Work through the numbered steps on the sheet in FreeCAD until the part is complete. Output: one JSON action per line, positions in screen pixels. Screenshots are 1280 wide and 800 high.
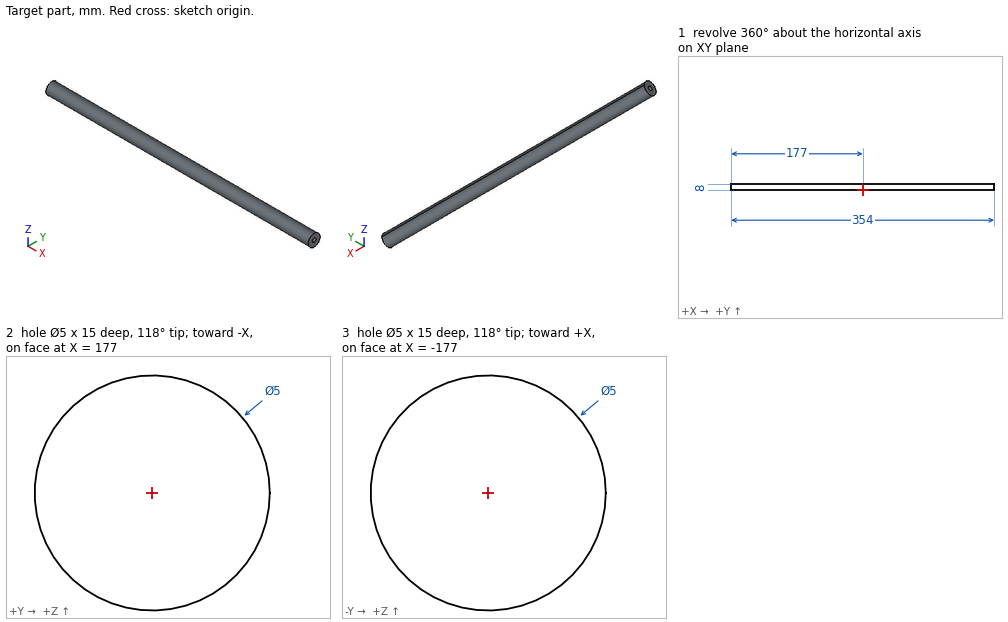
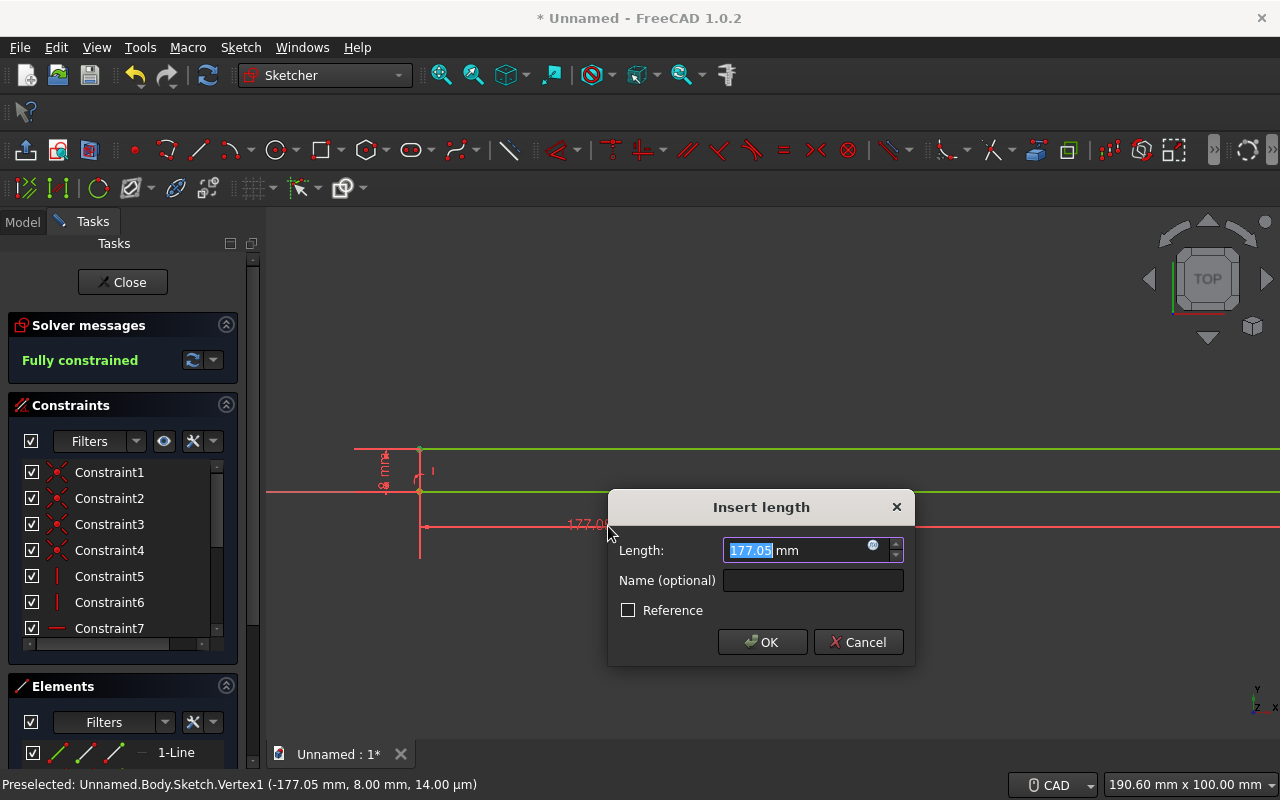
{"action": "type", "text": "177"}
{"action": "key", "text": "Return"}
{"action": "key", "text": "Escape"}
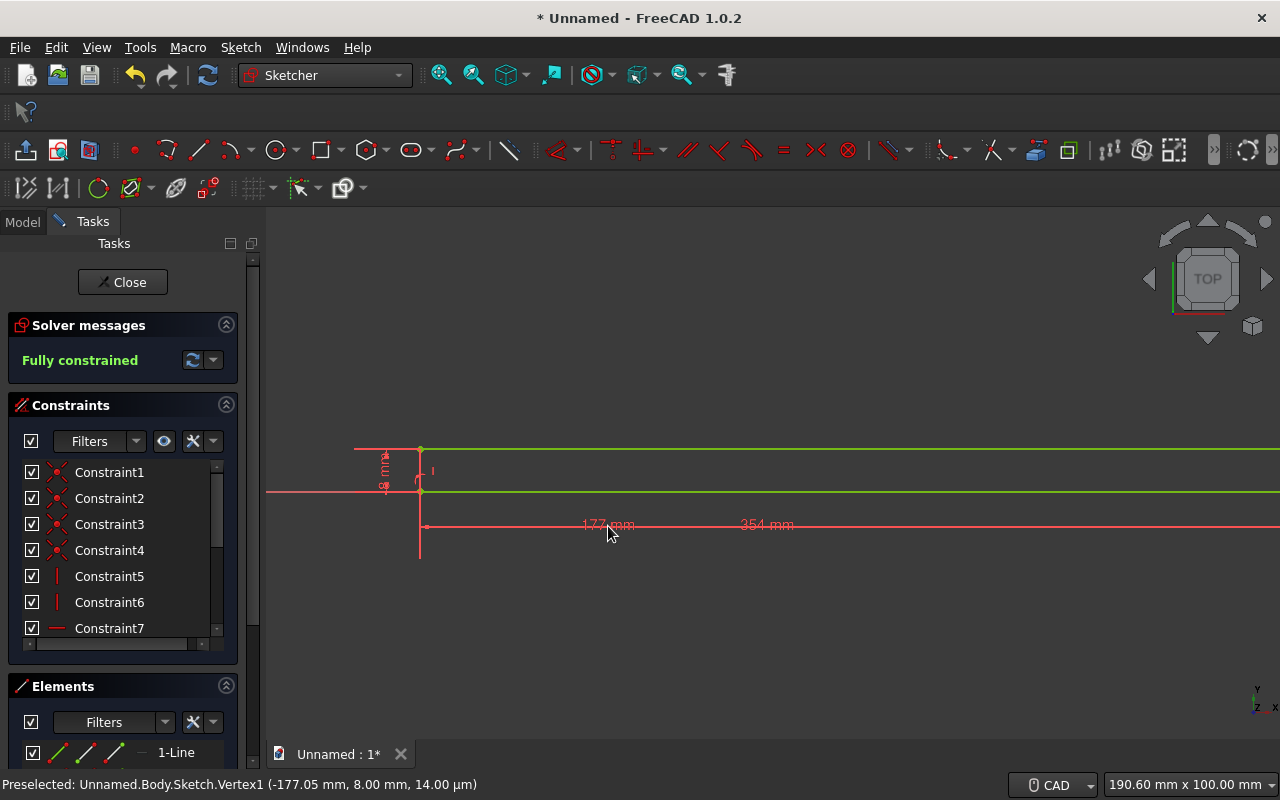
{"action": "left_click", "coordinate": [123, 282]}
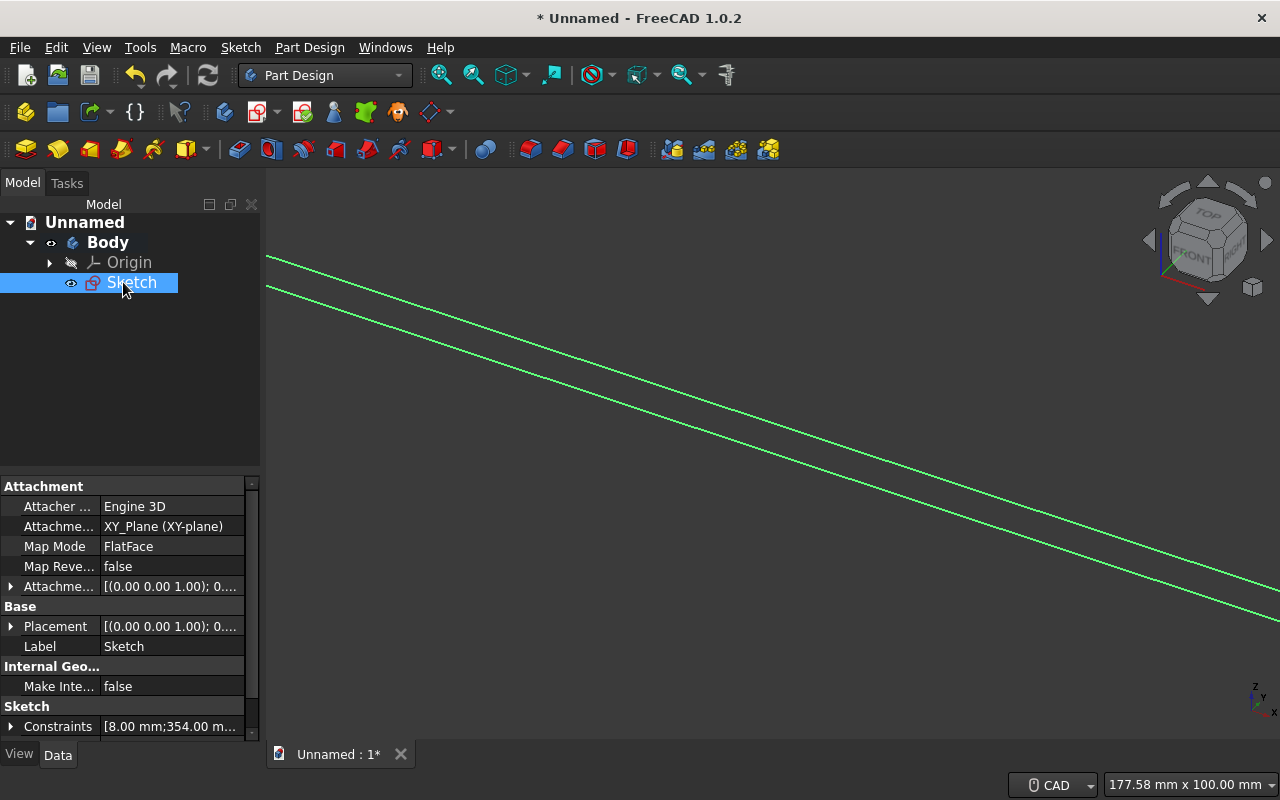
{"action": "left_click", "coordinate": [58, 150]}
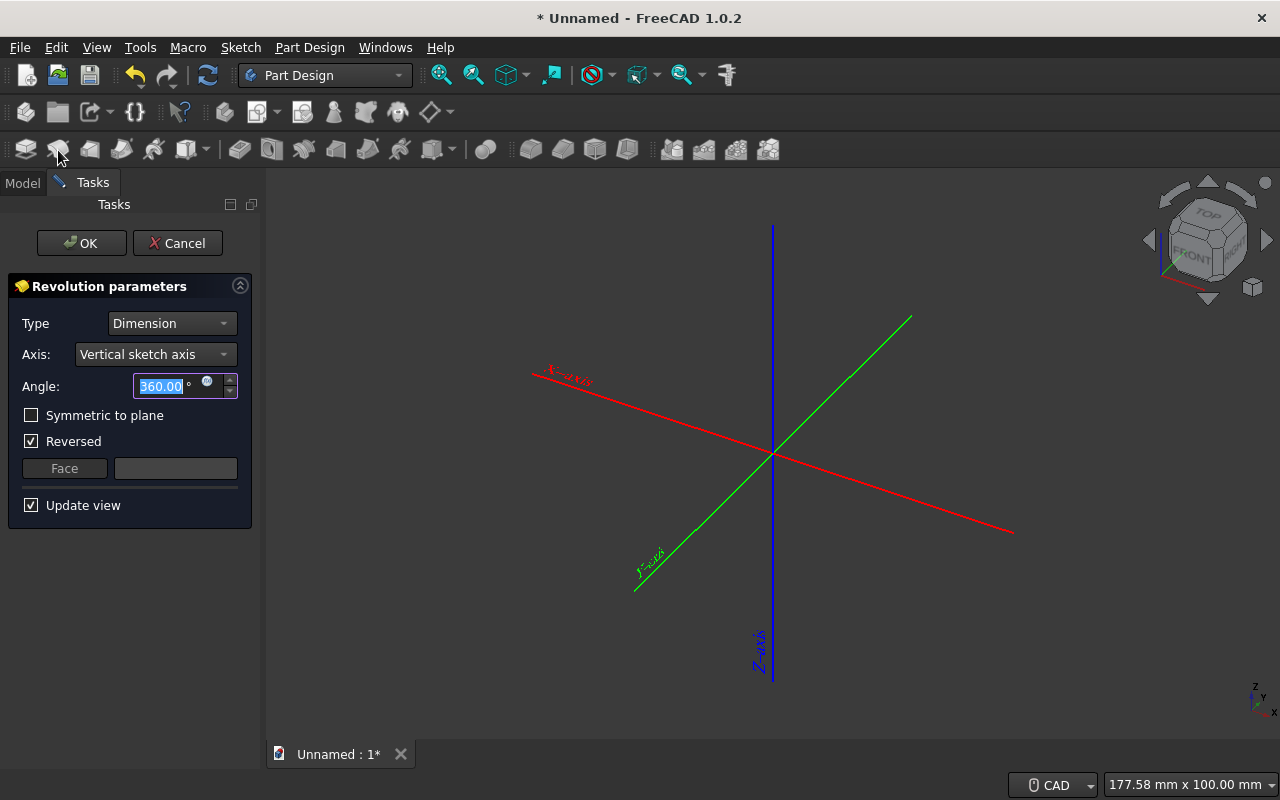
{"action": "left_click", "coordinate": [156, 354]}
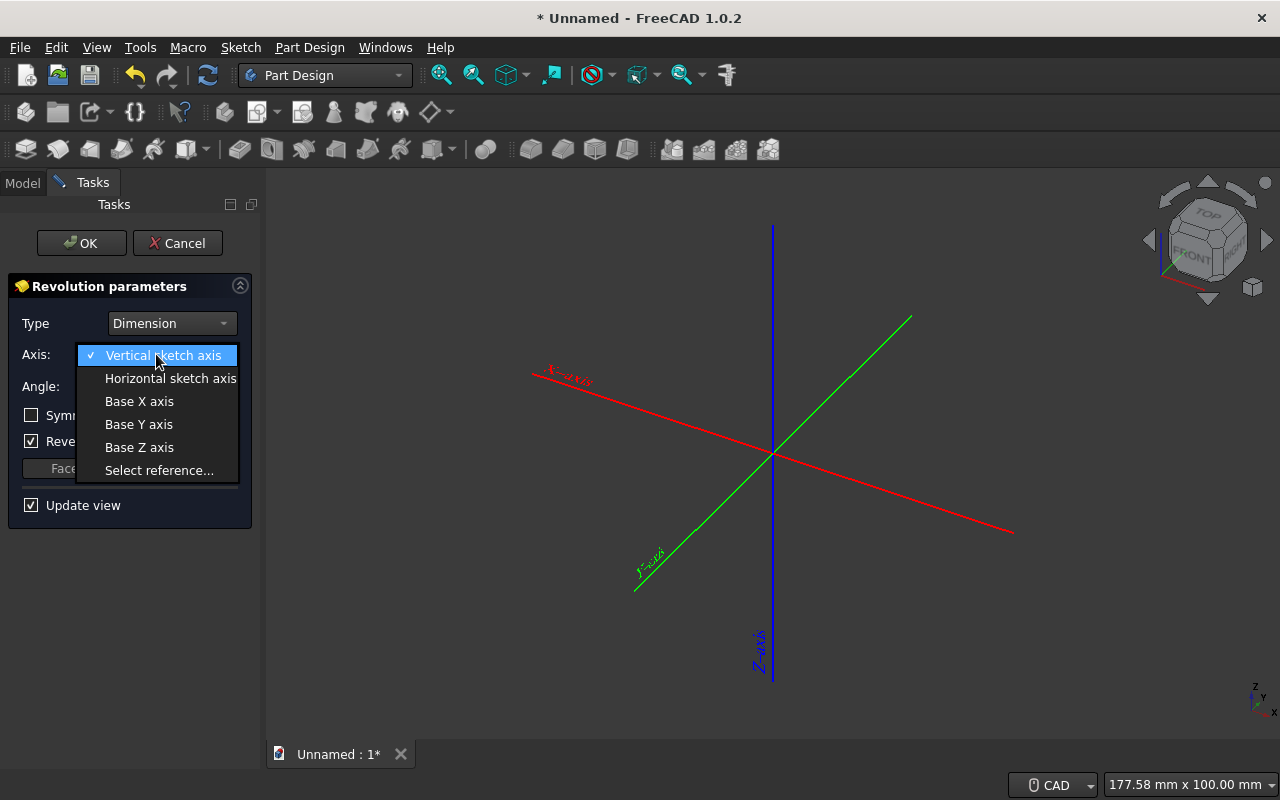
{"action": "left_click", "coordinate": [156, 378]}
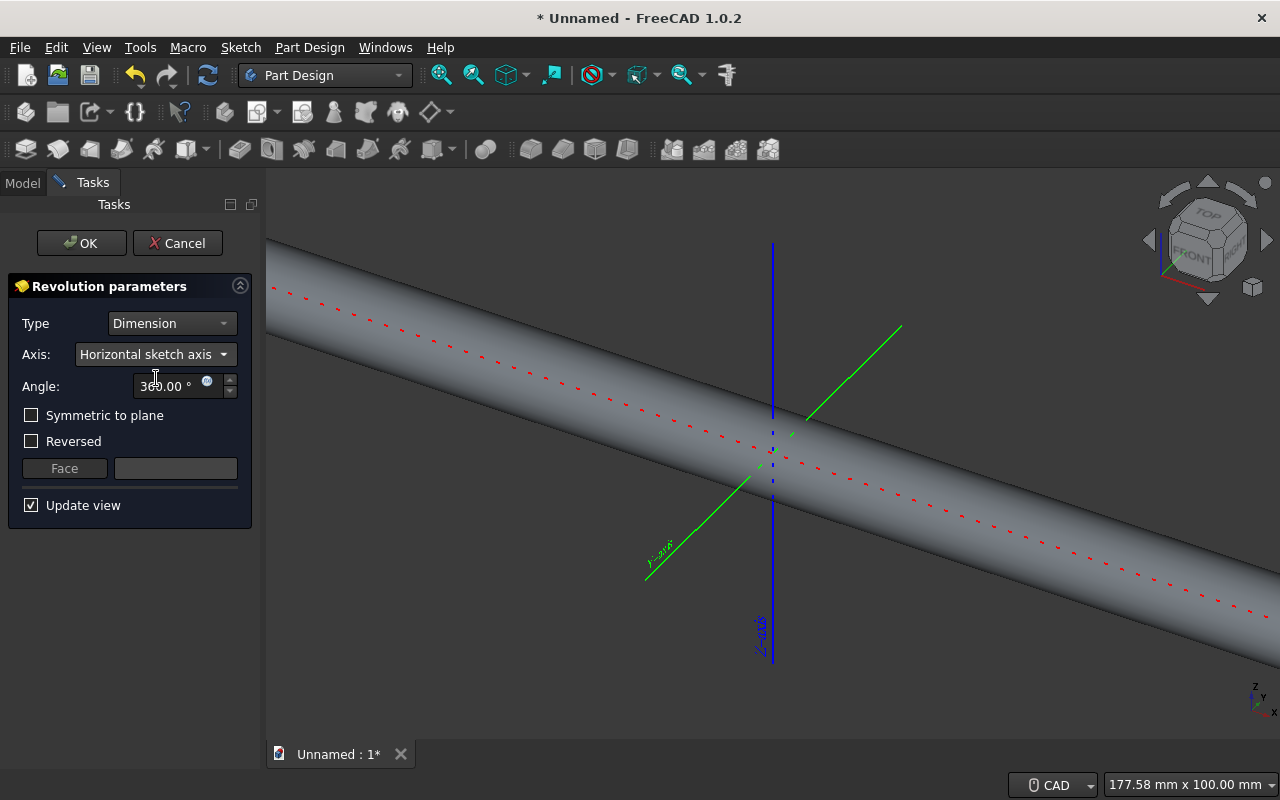
{"action": "left_click", "coordinate": [82, 243]}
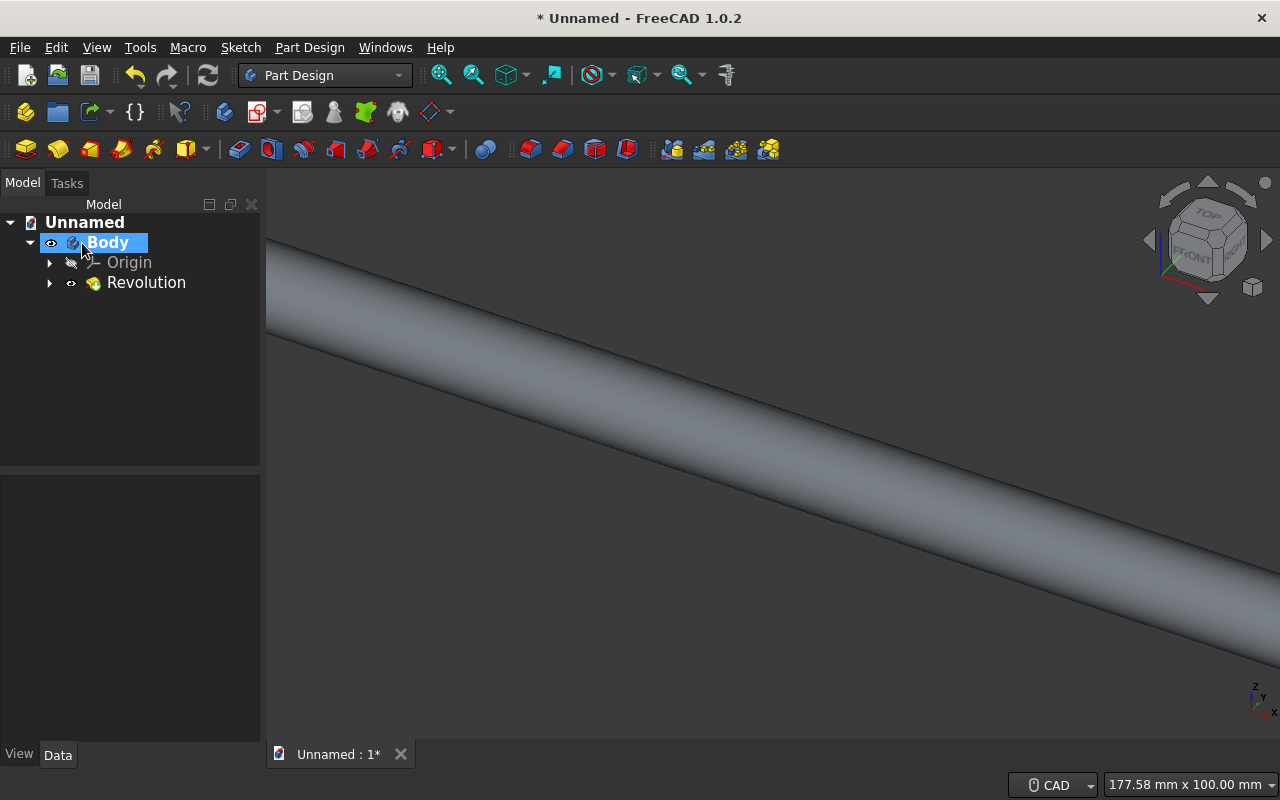
{"action": "left_click", "coordinate": [442, 76]}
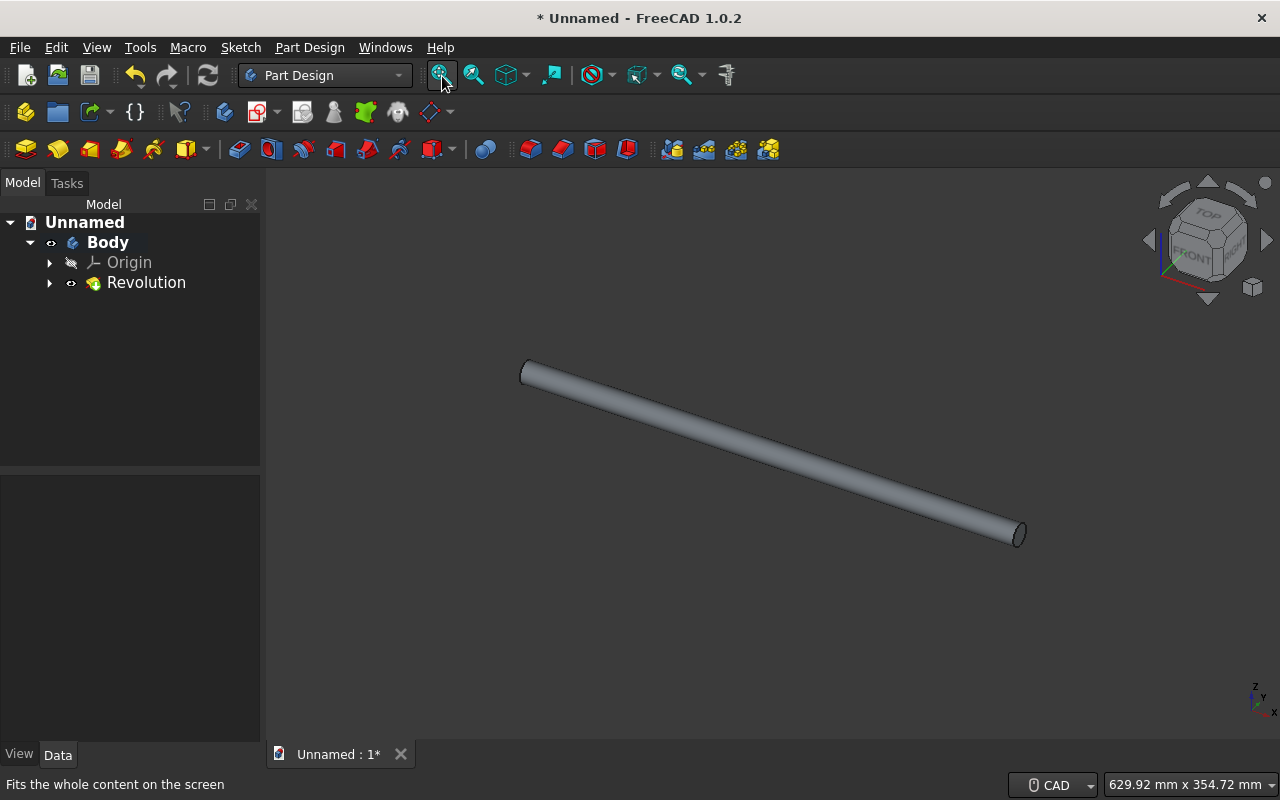
{"action": "key", "text": "0"}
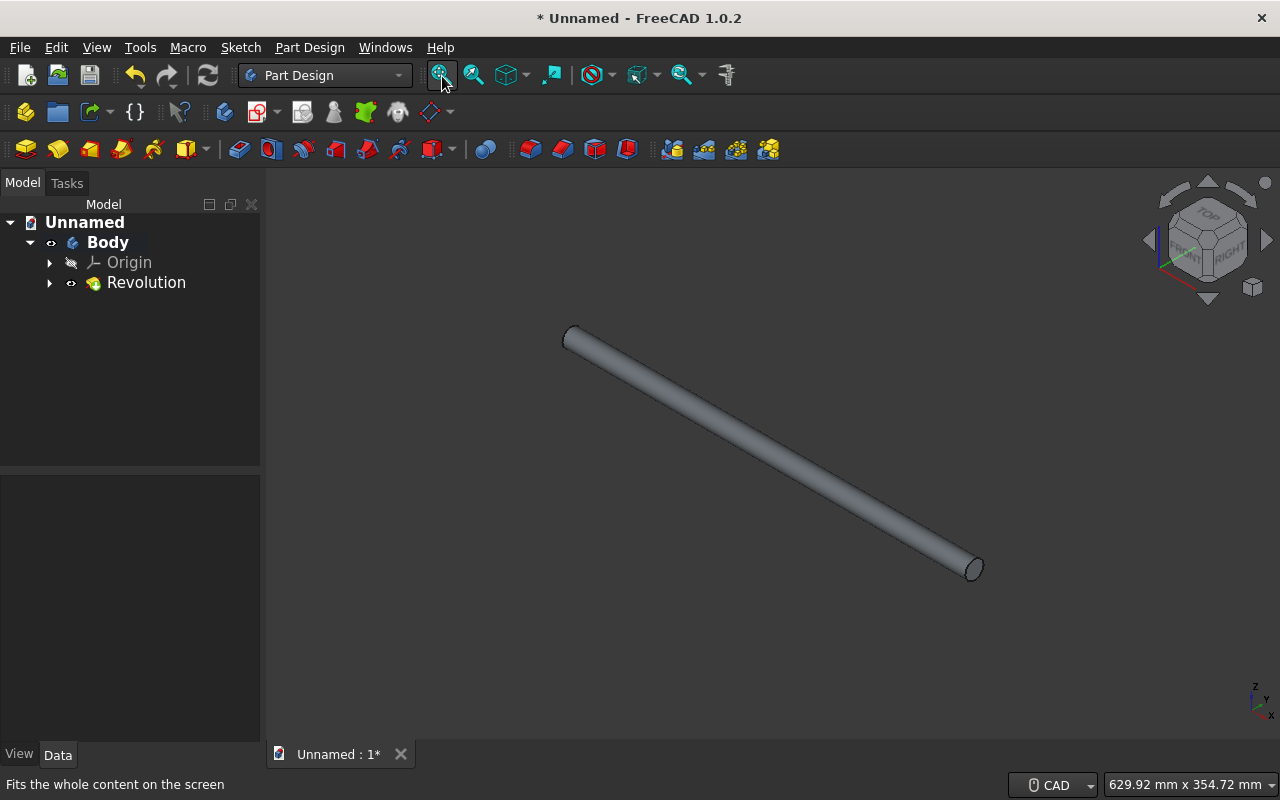
{"action": "key", "text": "3"}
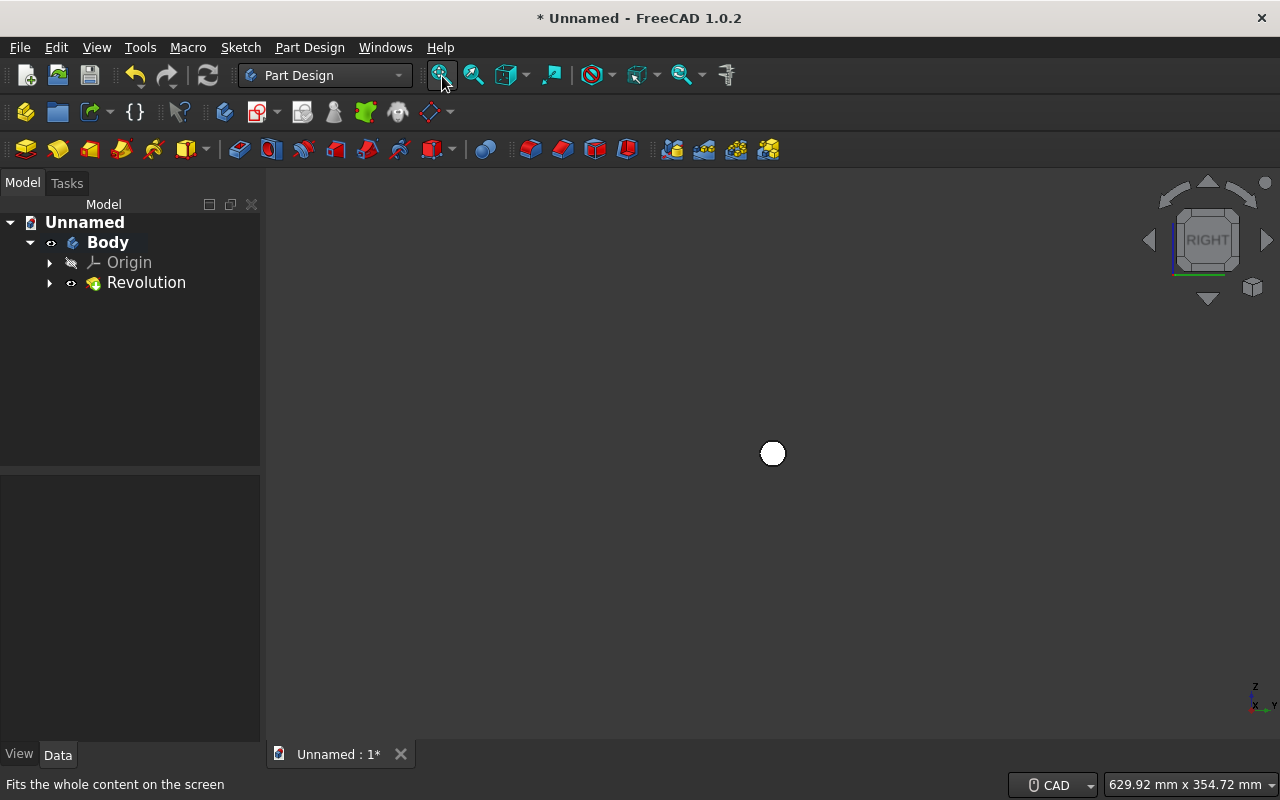
{"action": "key", "text": "v f"}